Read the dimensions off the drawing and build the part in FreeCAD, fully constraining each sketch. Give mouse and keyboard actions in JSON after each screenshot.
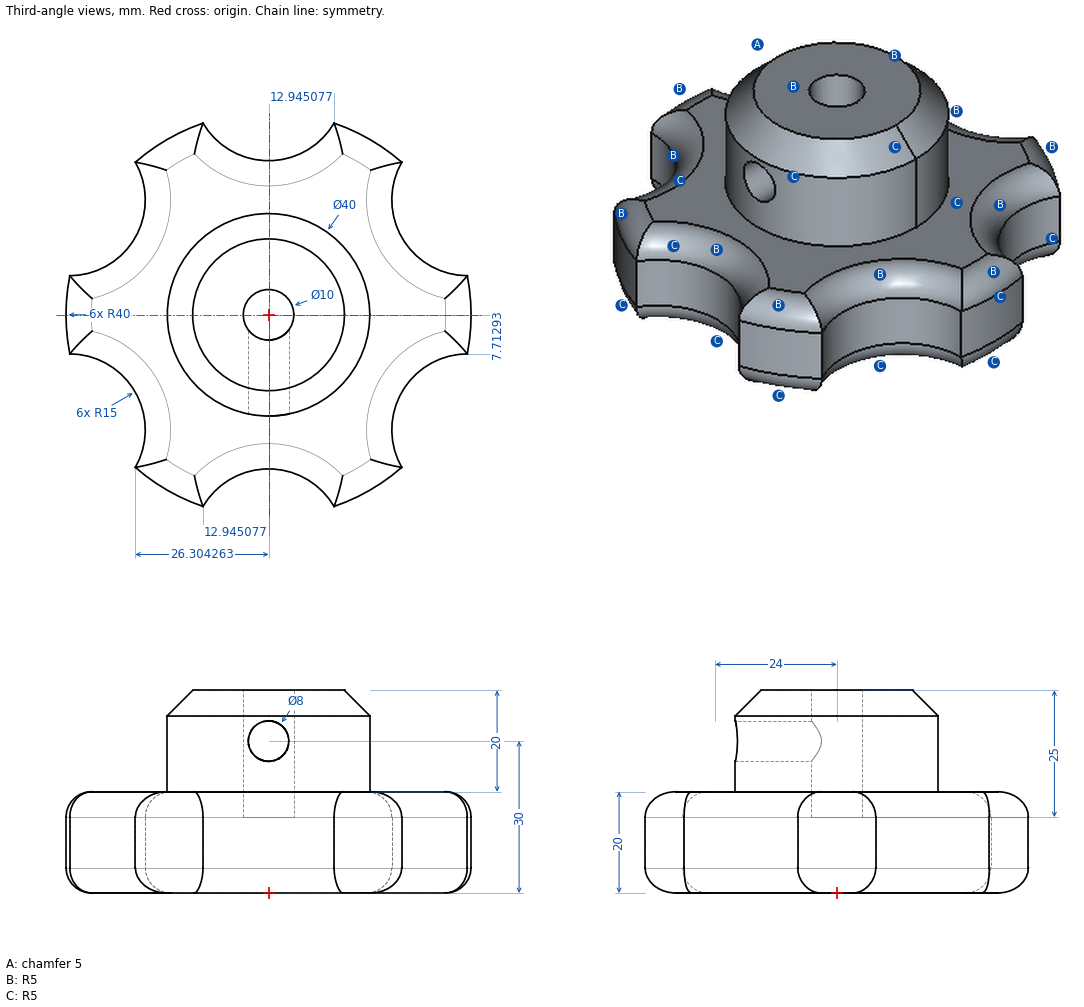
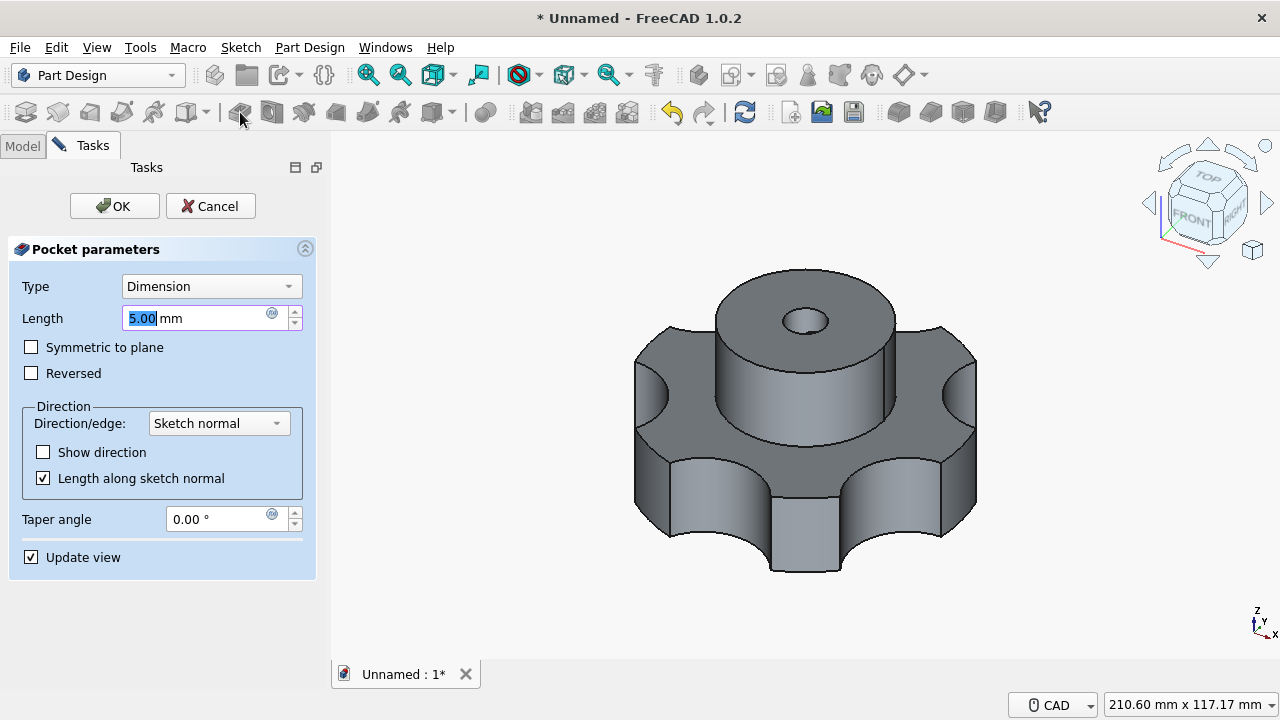
{"action": "type", "text": "24"}
{"action": "key", "text": "Tab"}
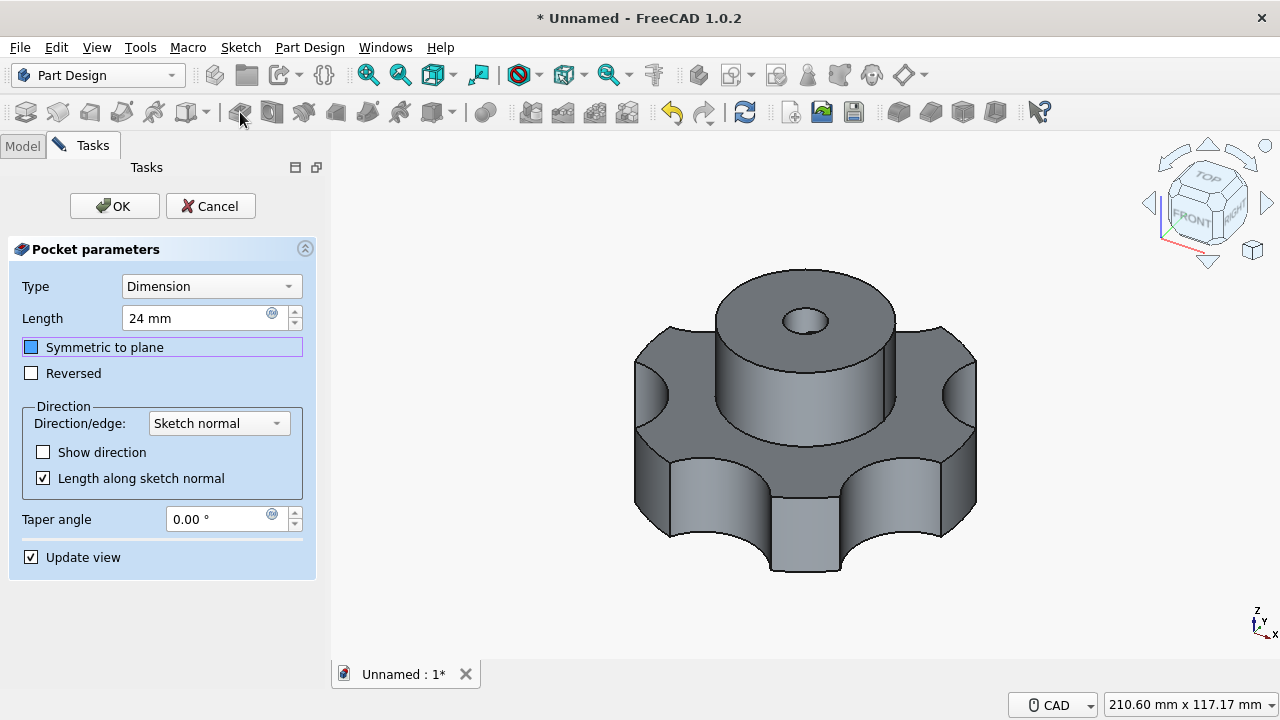
{"action": "left_click", "coordinate": [30, 373]}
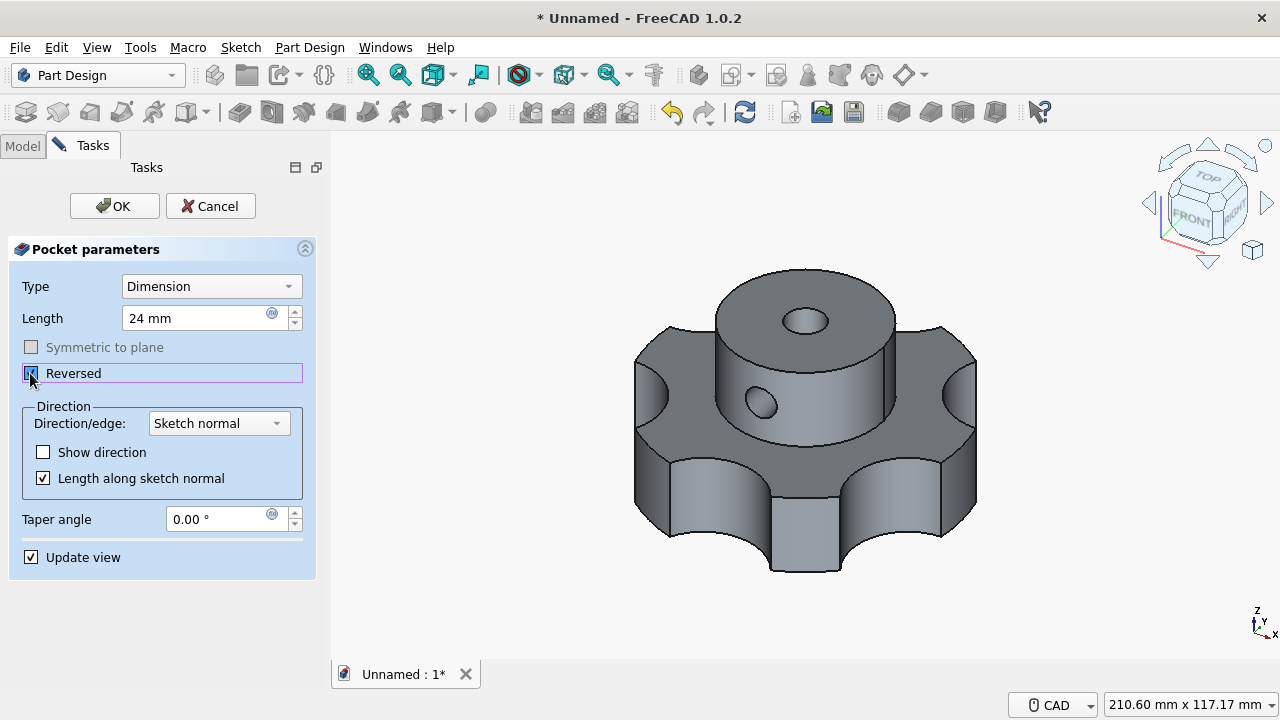
{"action": "left_click", "coordinate": [115, 206]}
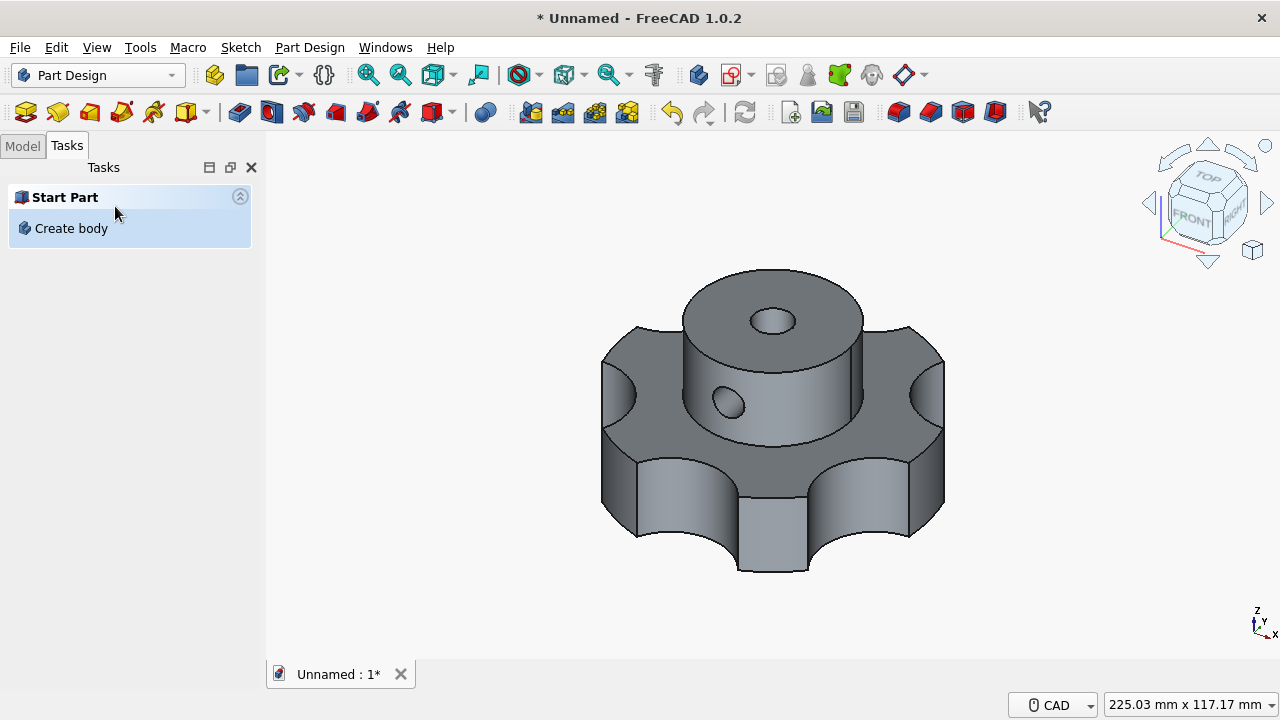
{"action": "left_click", "coordinate": [683, 326]}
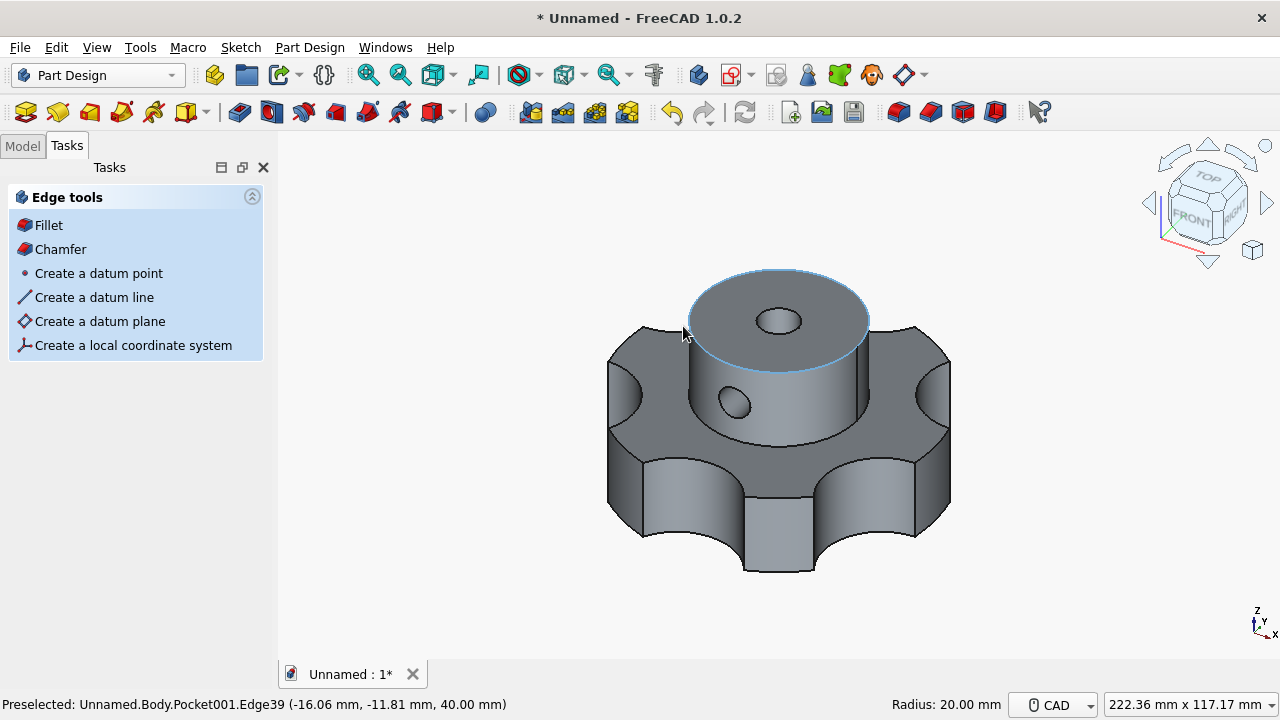
{"action": "left_click", "coordinate": [932, 112]}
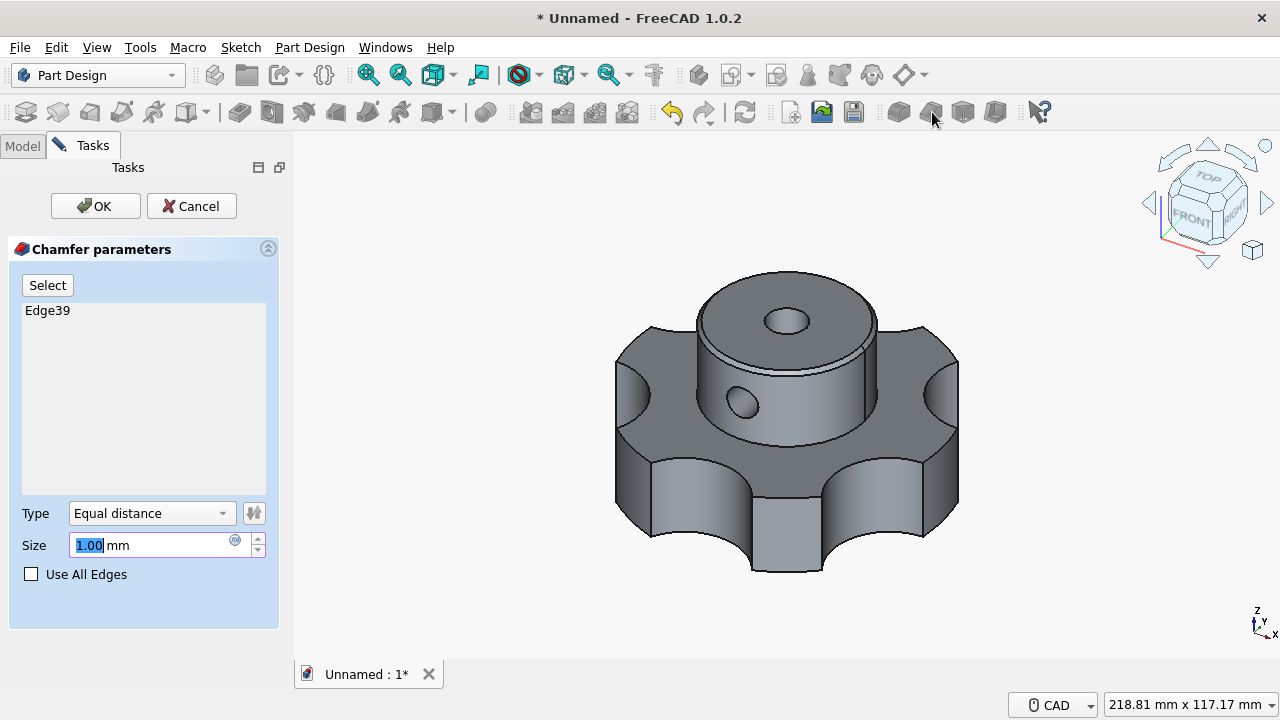
{"action": "type", "text": "5"}
{"action": "key", "text": "Tab"}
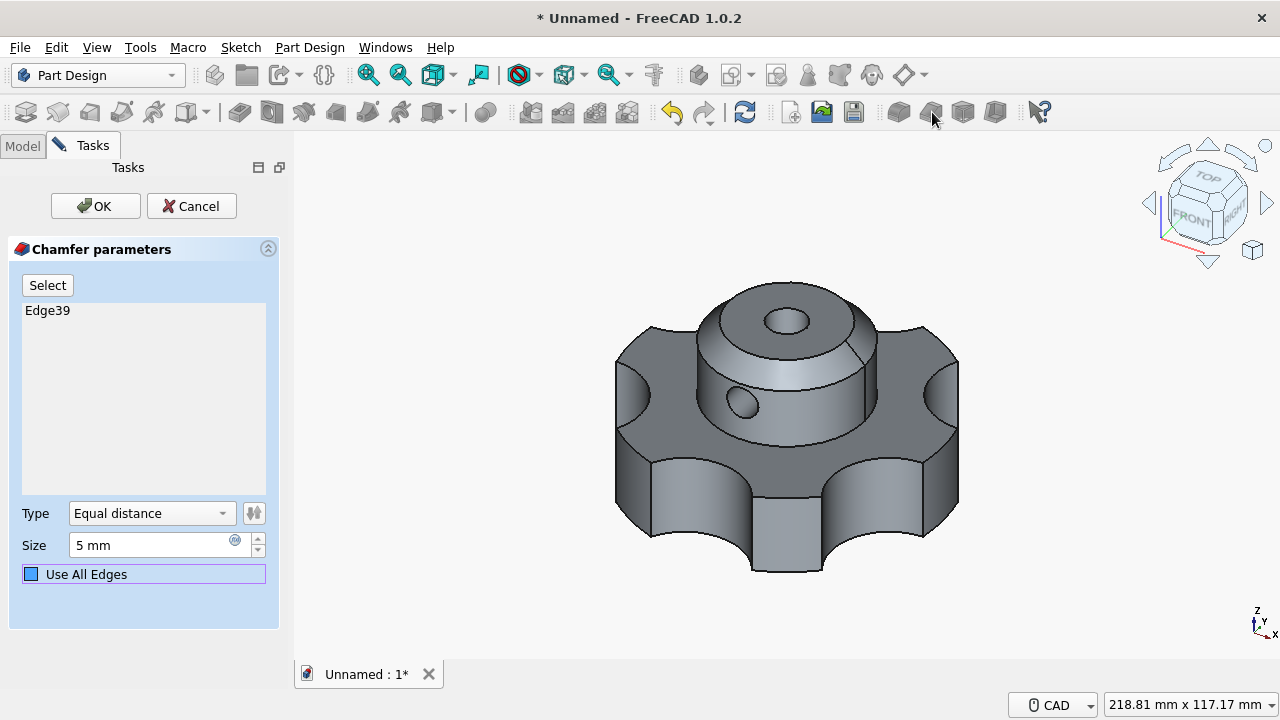
{"action": "left_click", "coordinate": [96, 206]}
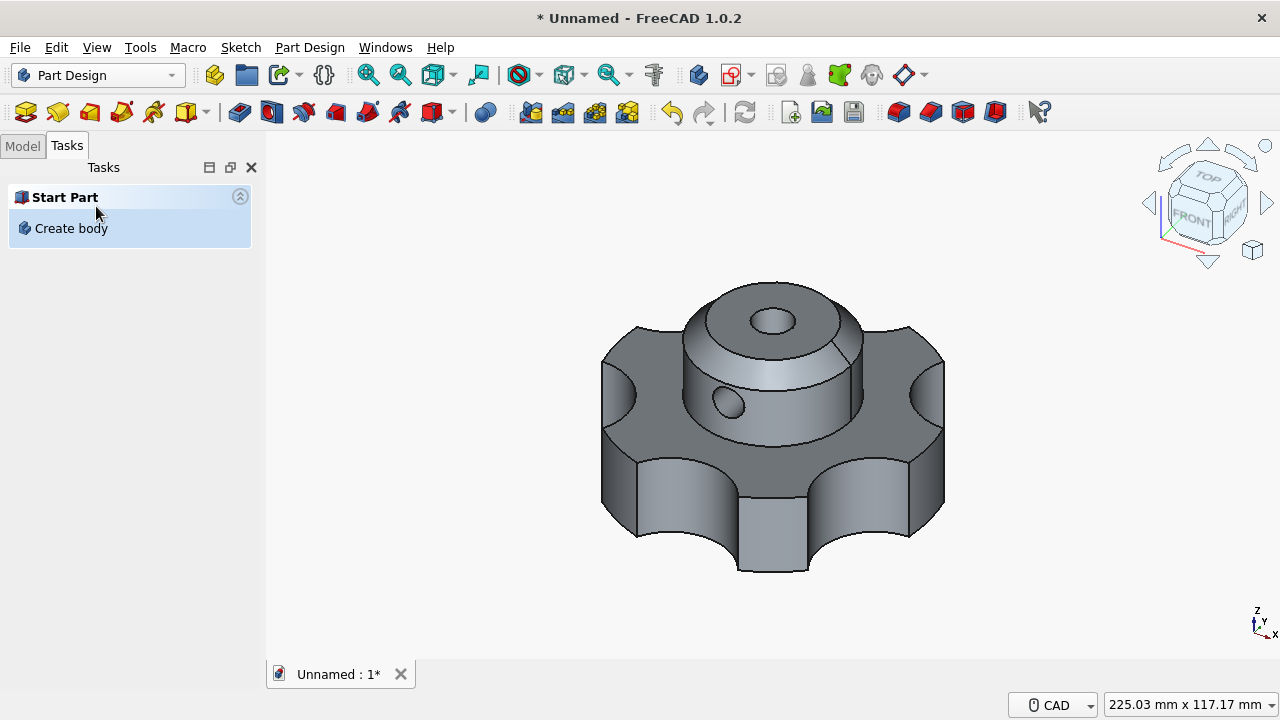
{"action": "left_click", "coordinate": [610, 349]}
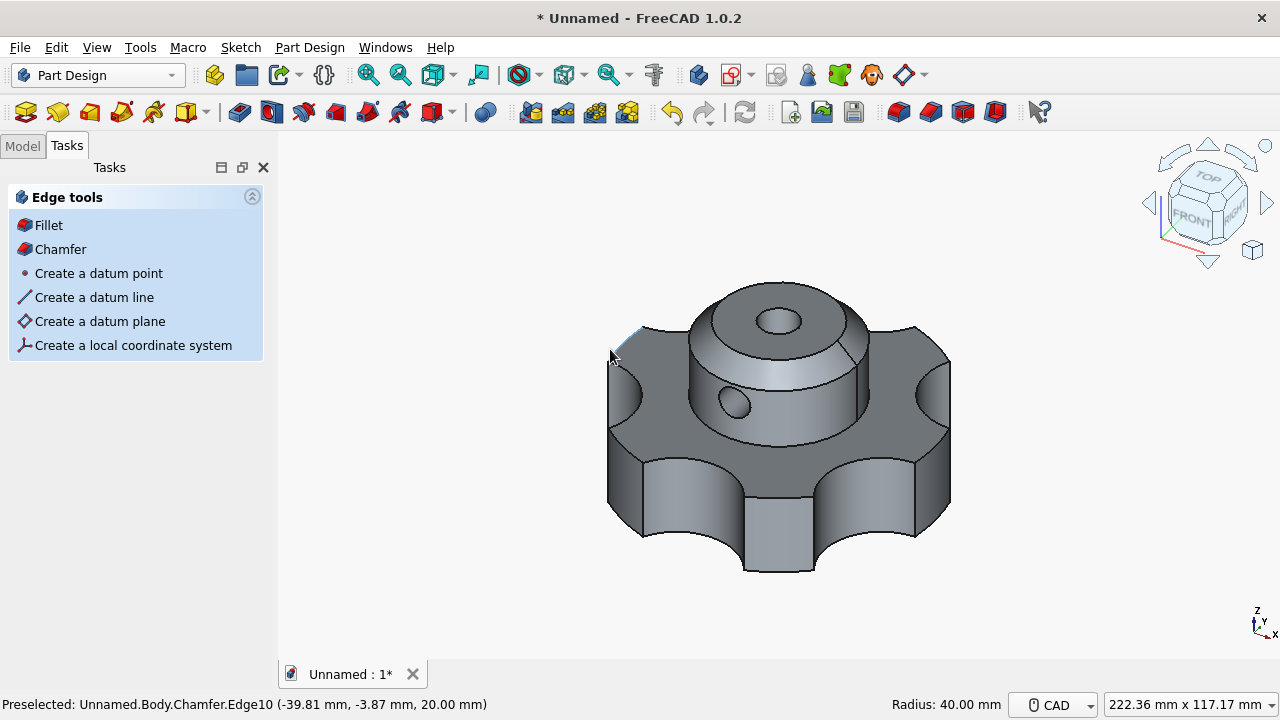
{"action": "left_click", "coordinate": [640, 386], "text": "ctrl"}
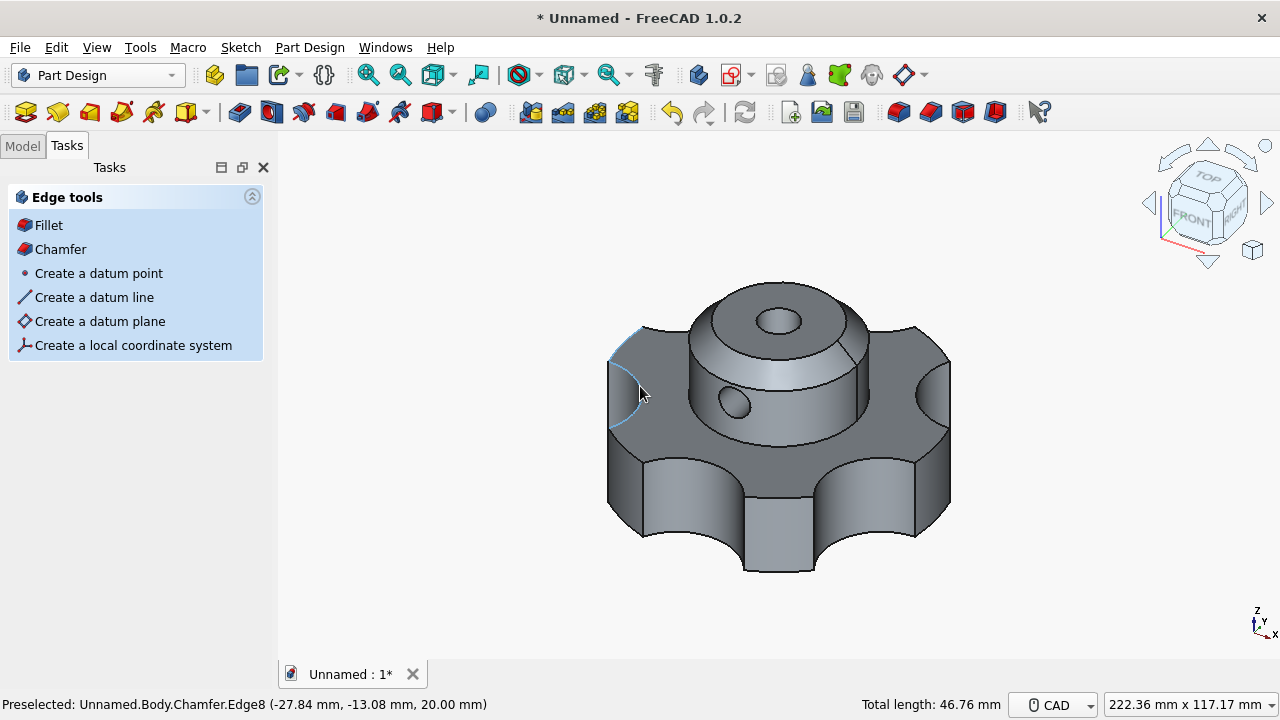
{"action": "left_click", "coordinate": [623, 446], "text": "ctrl"}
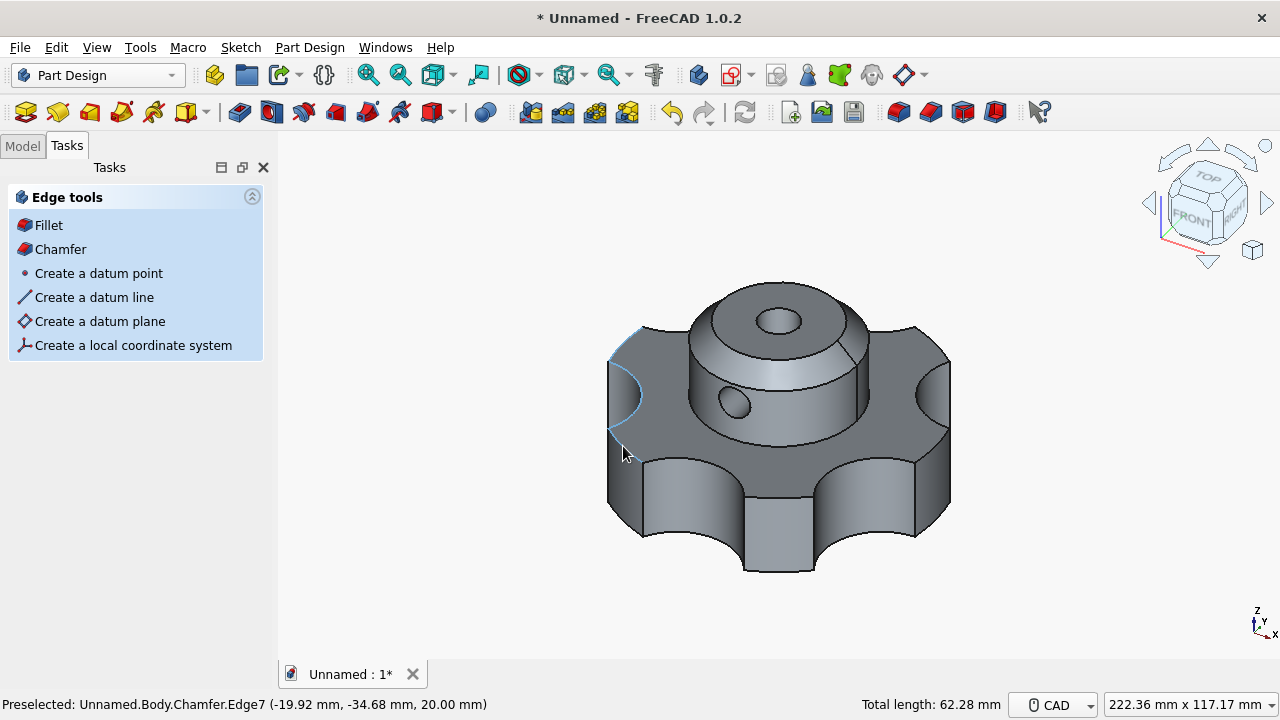
{"action": "left_click", "coordinate": [710, 462], "text": "ctrl"}